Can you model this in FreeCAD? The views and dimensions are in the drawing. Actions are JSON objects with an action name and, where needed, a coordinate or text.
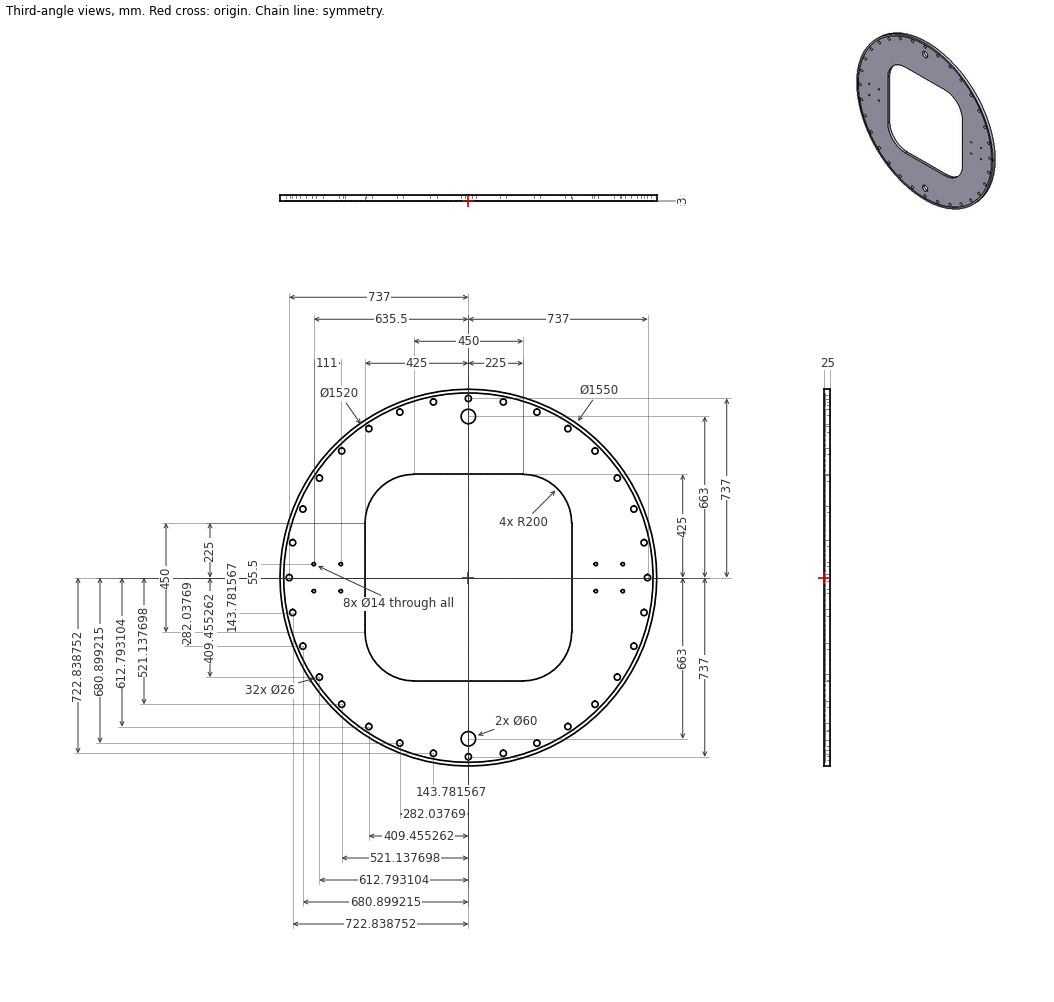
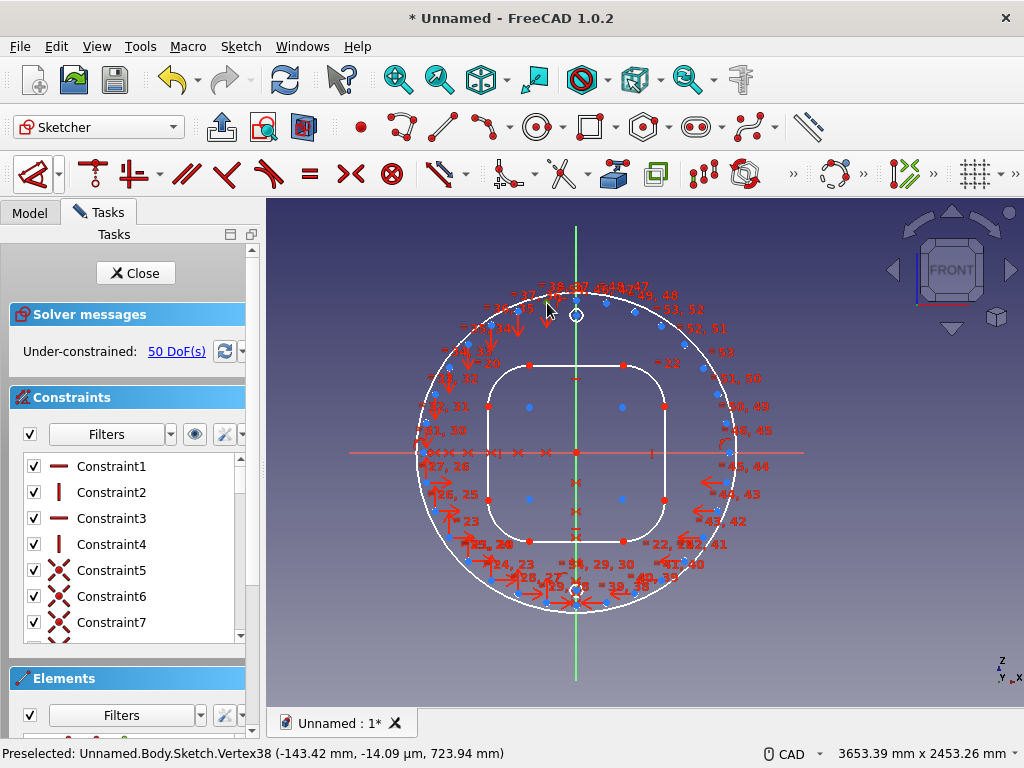
{"action": "scroll", "coordinate": [606, 303], "scroll_direction": "up", "scroll_amount": 4}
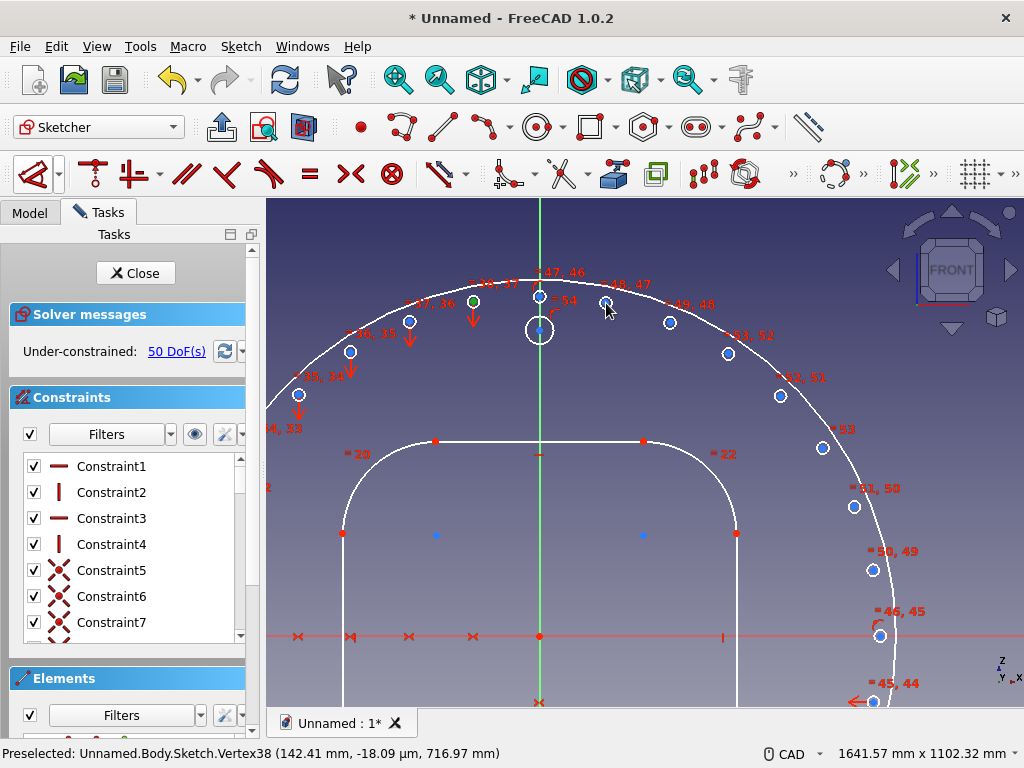
{"action": "left_click", "coordinate": [606, 303]}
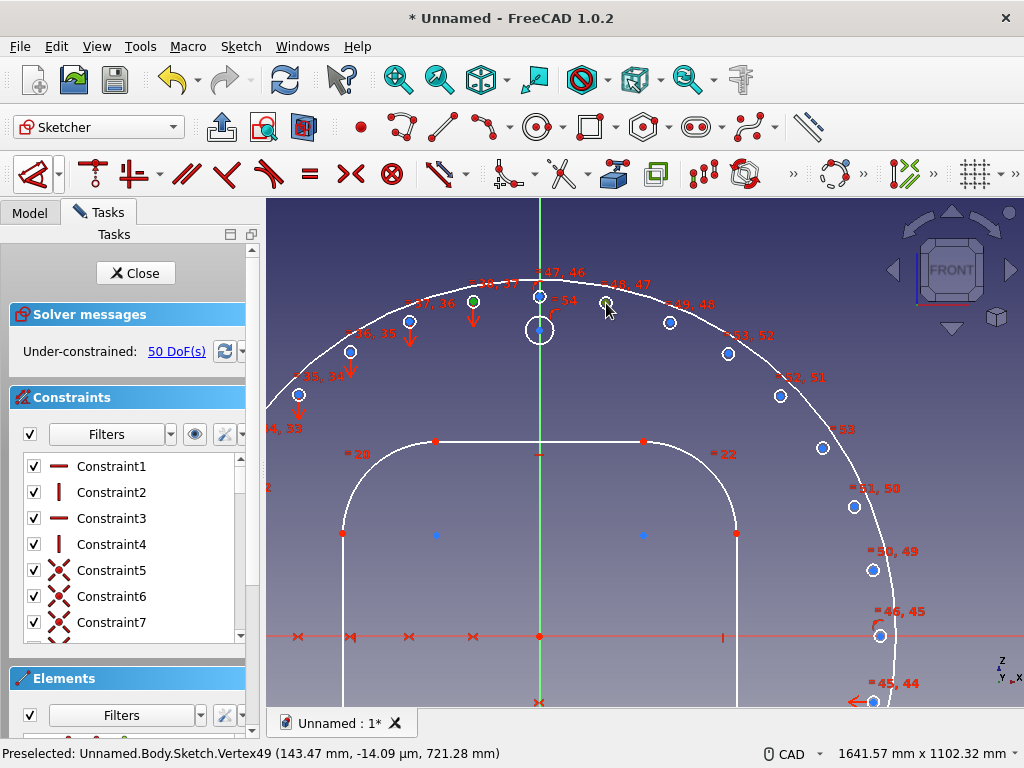
{"action": "left_click", "coordinate": [540, 582]}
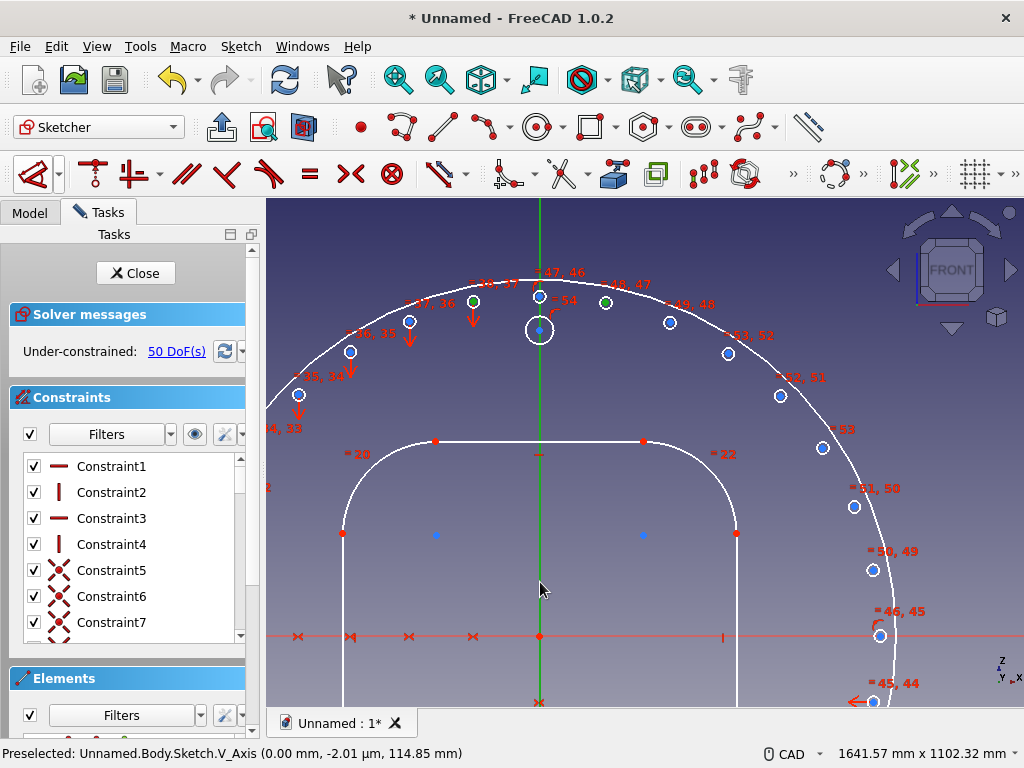
{"action": "left_click", "coordinate": [351, 174]}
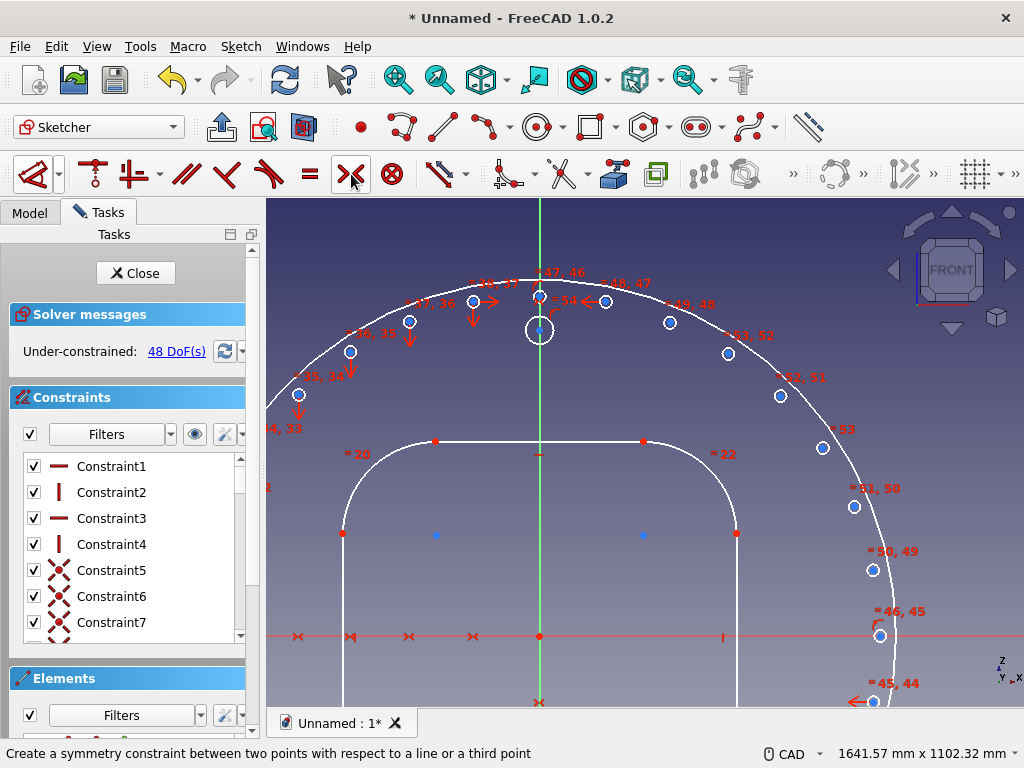
{"action": "left_click", "coordinate": [410, 322]}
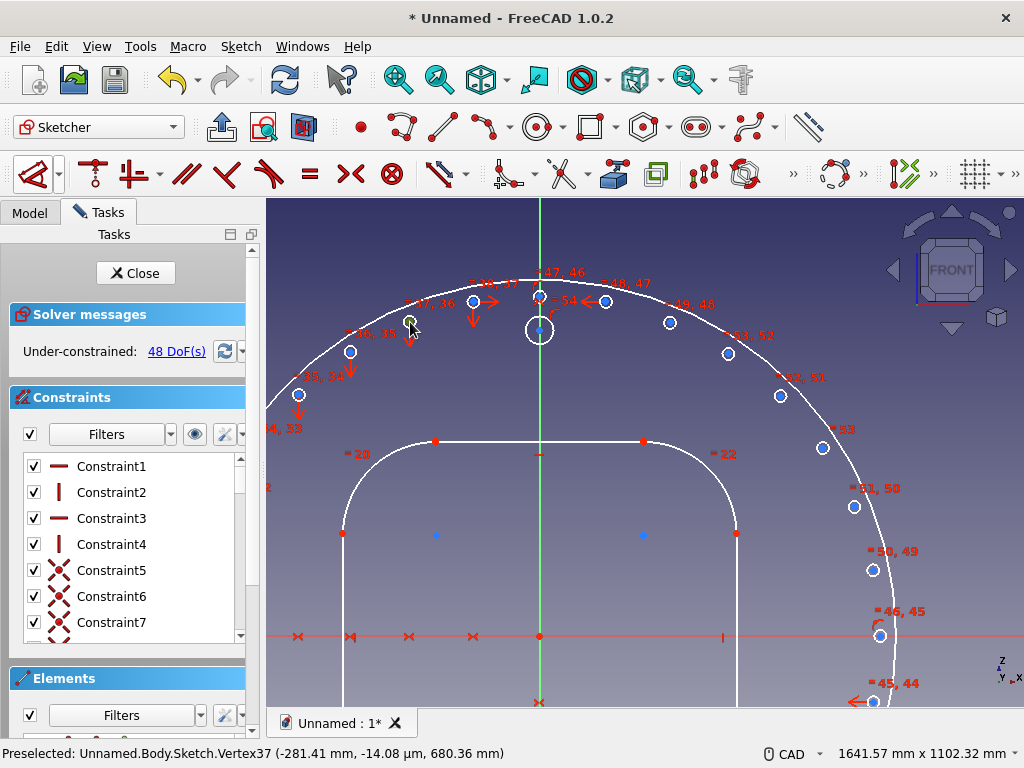
{"action": "left_click", "coordinate": [670, 323]}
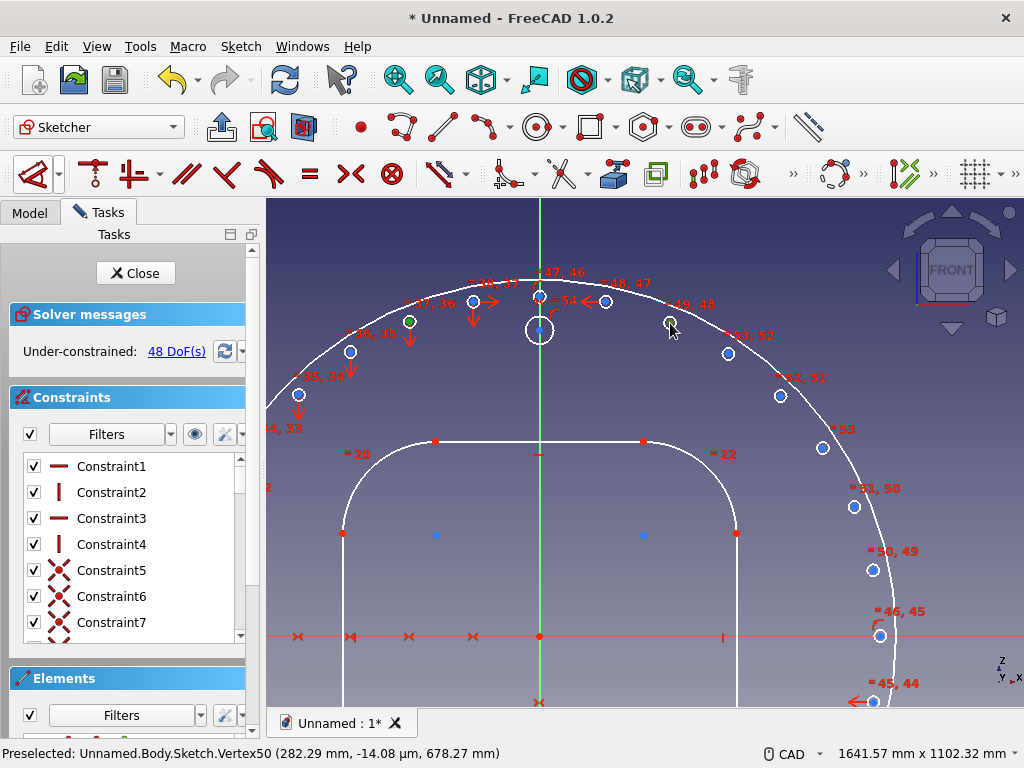
{"action": "left_click", "coordinate": [540, 582]}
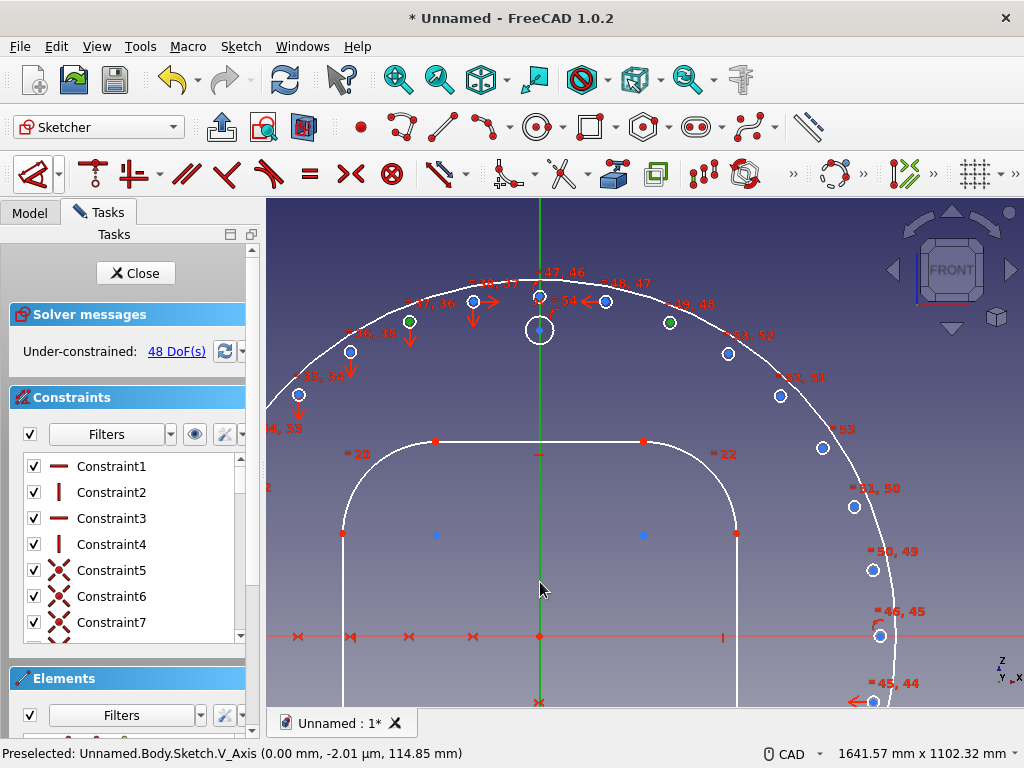
{"action": "left_click", "coordinate": [351, 174]}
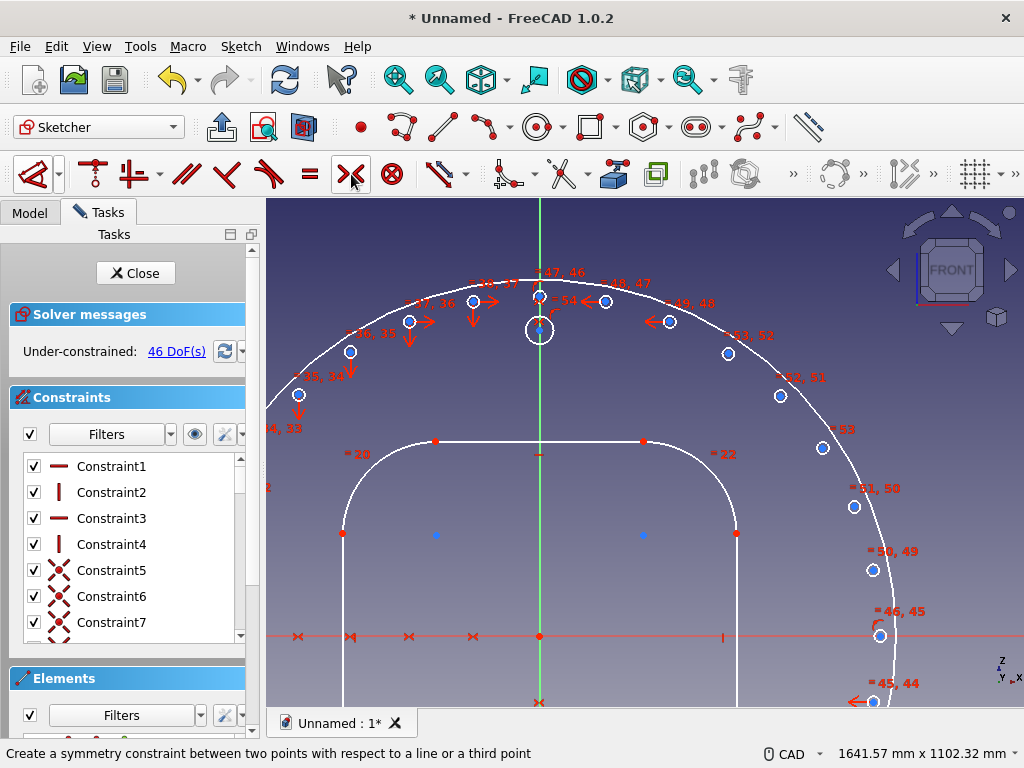
{"action": "scroll", "coordinate": [607, 303], "scroll_direction": "down", "scroll_amount": 4}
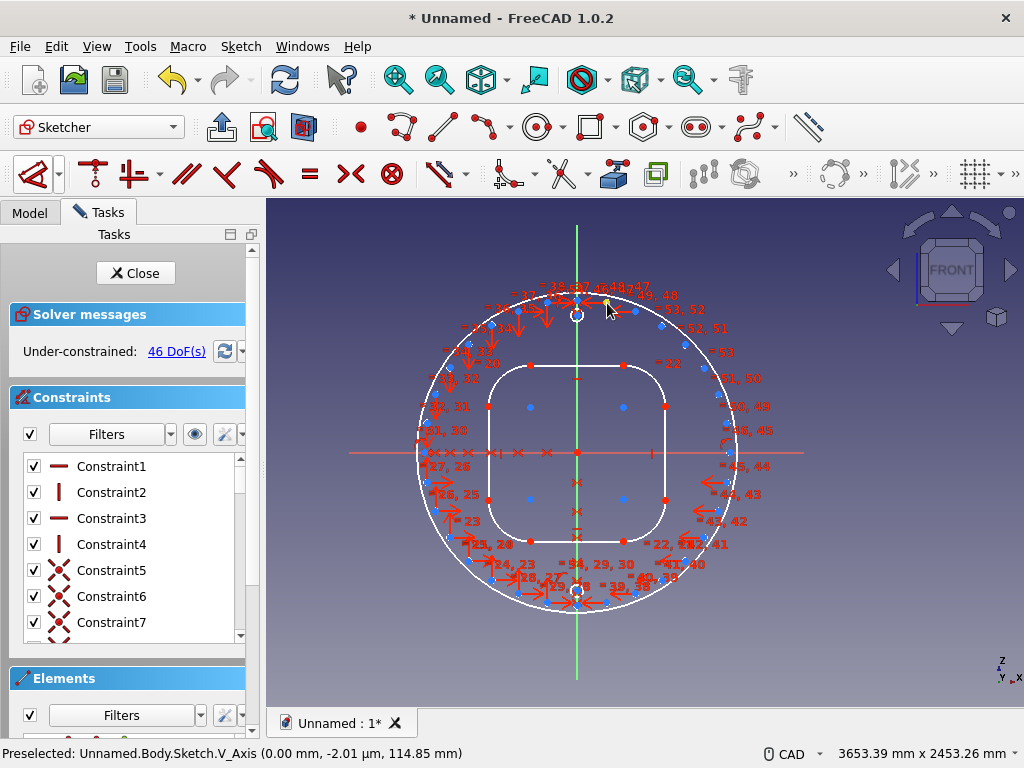
{"action": "left_click", "coordinate": [427, 423]}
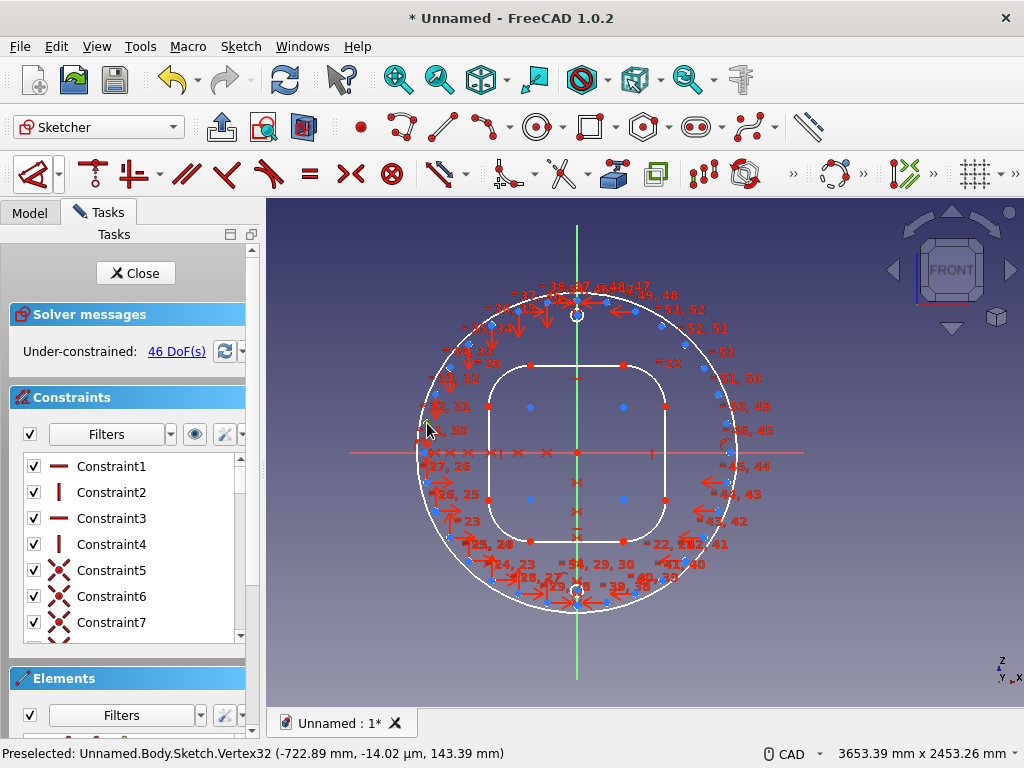
{"action": "left_click", "coordinate": [727, 423]}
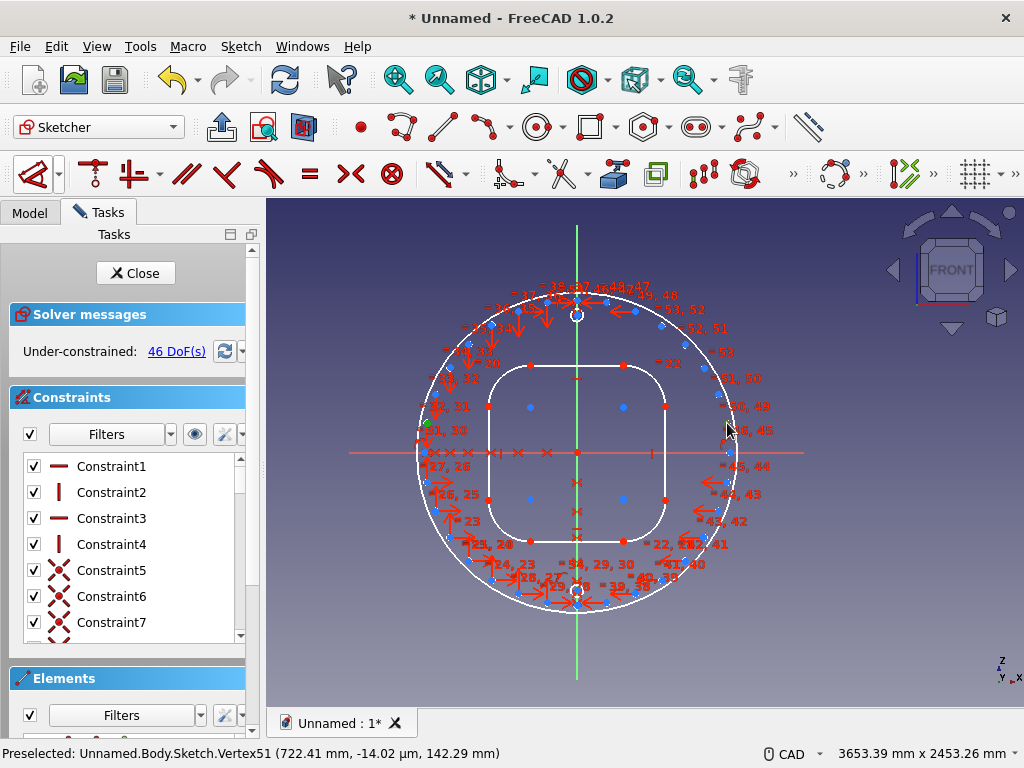
{"action": "left_click", "coordinate": [577, 647]}